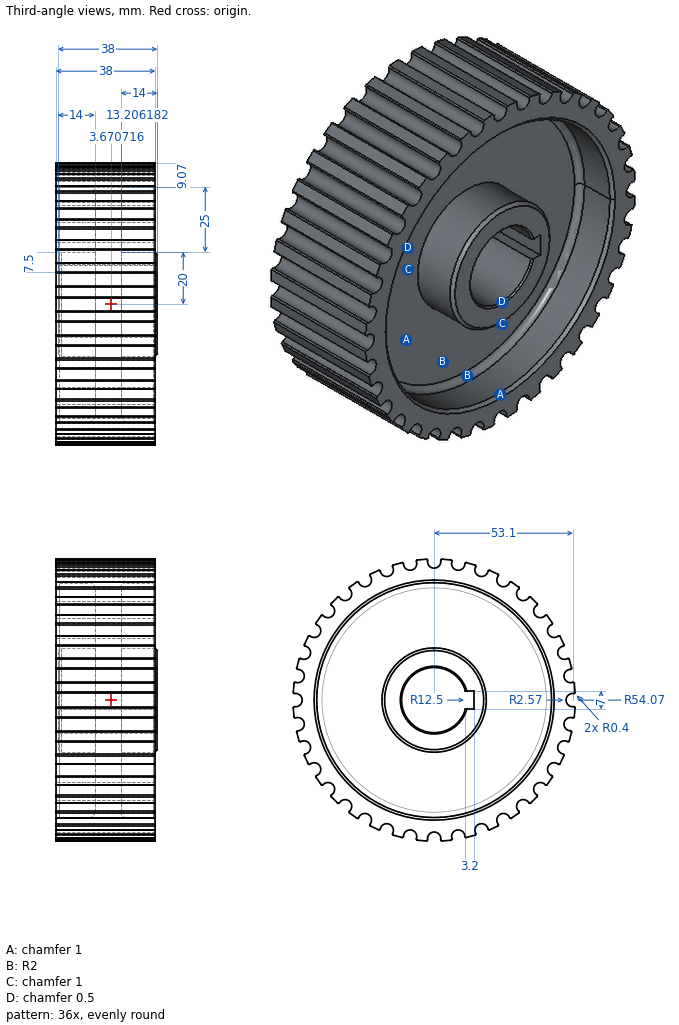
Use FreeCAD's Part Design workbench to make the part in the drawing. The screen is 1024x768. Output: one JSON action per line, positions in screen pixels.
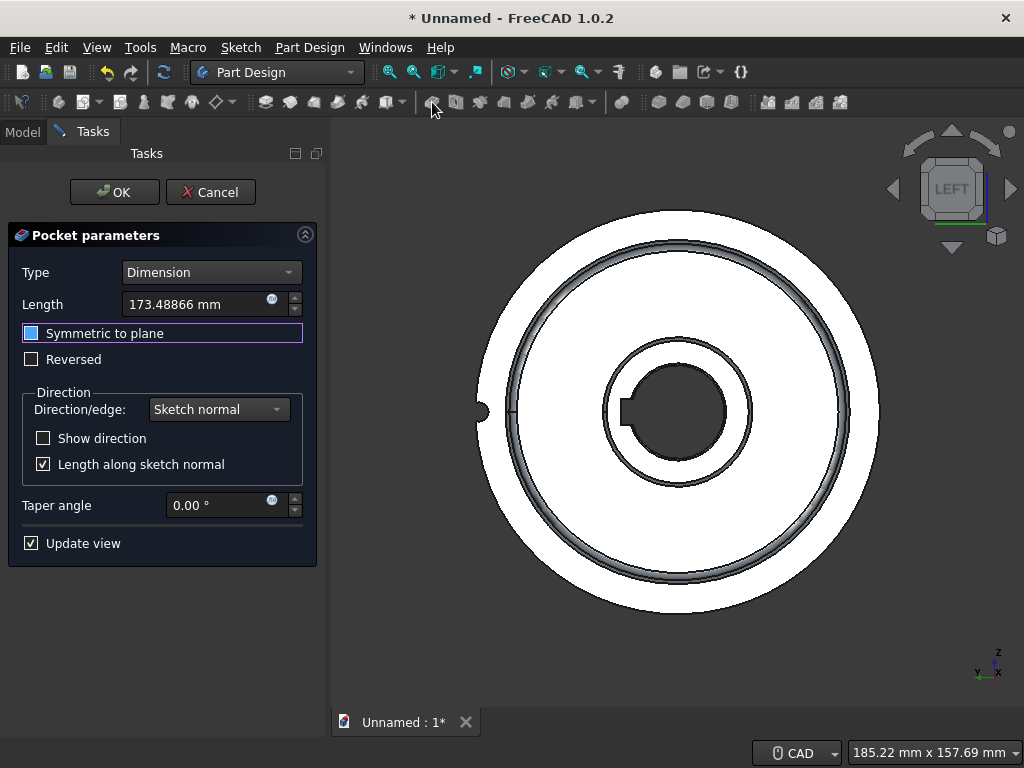
{"action": "left_click", "coordinate": [30, 333]}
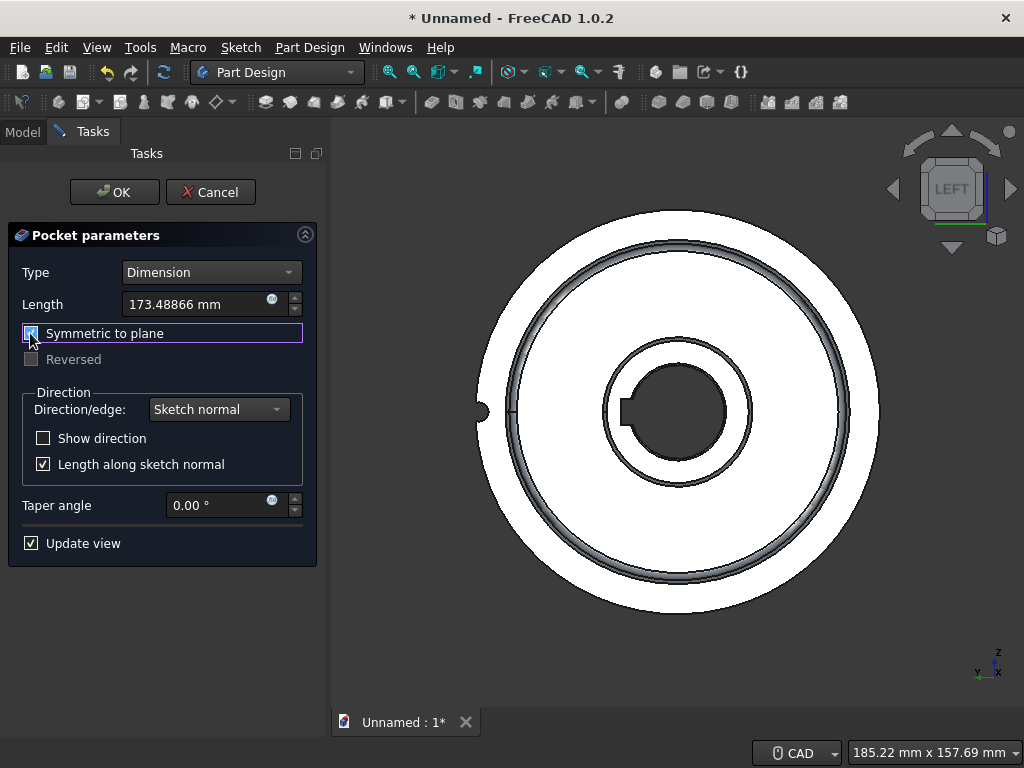
{"action": "left_click", "coordinate": [115, 192]}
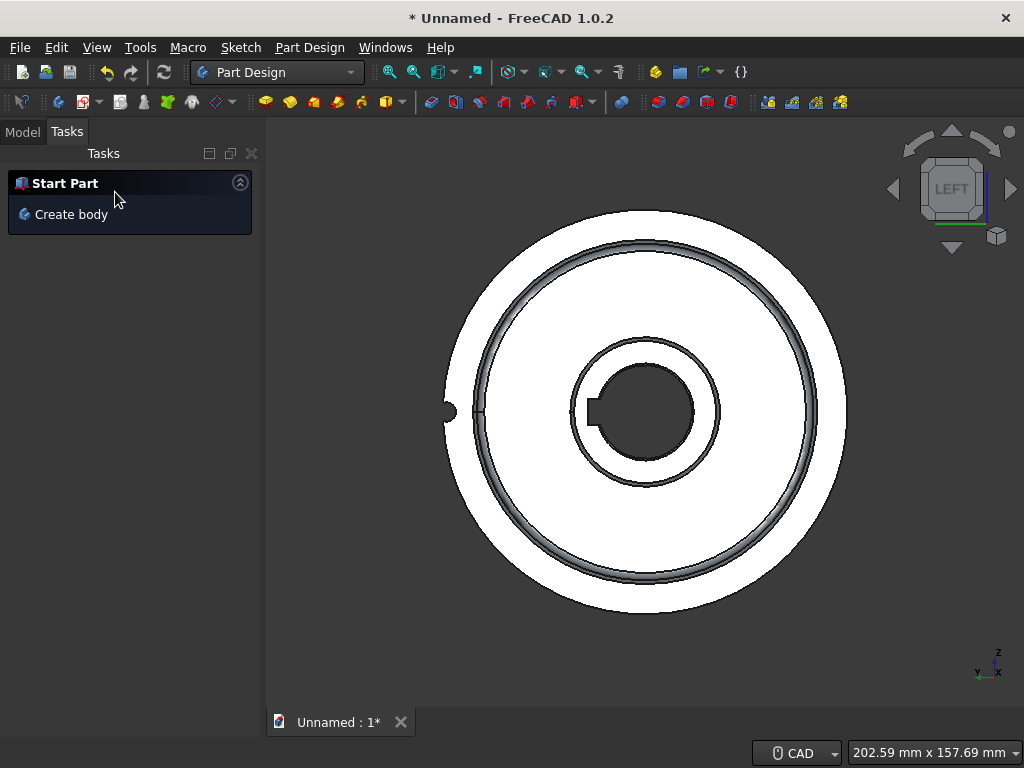
{"action": "left_click", "coordinate": [23, 131]}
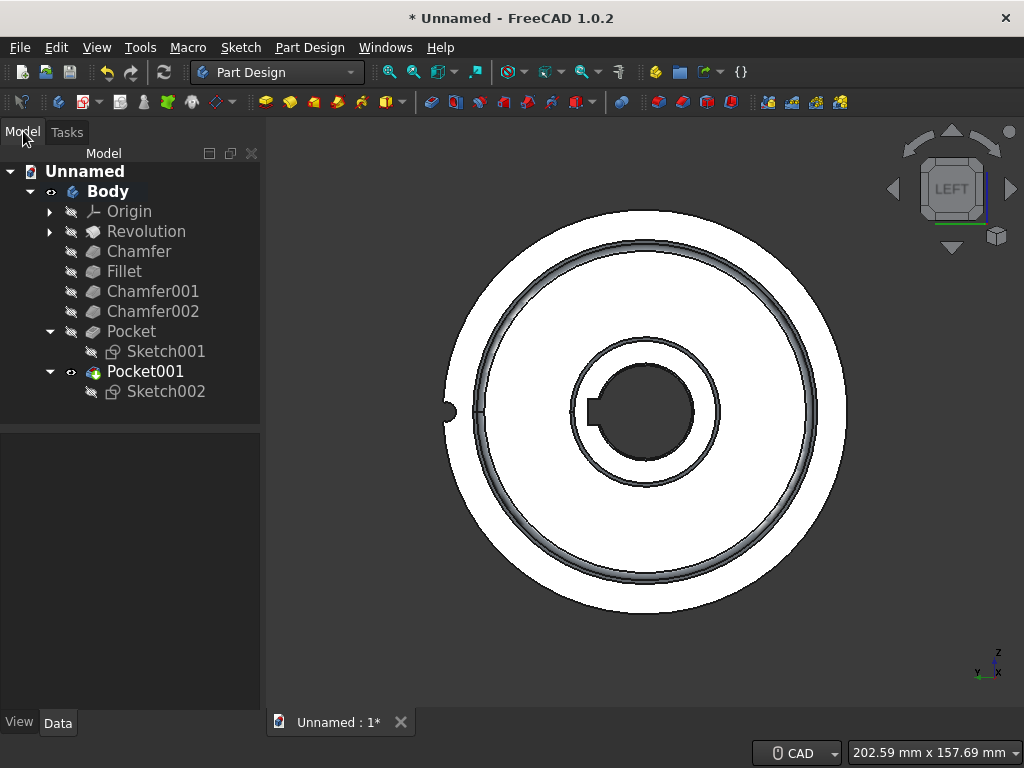
{"action": "left_click", "coordinate": [116, 372]}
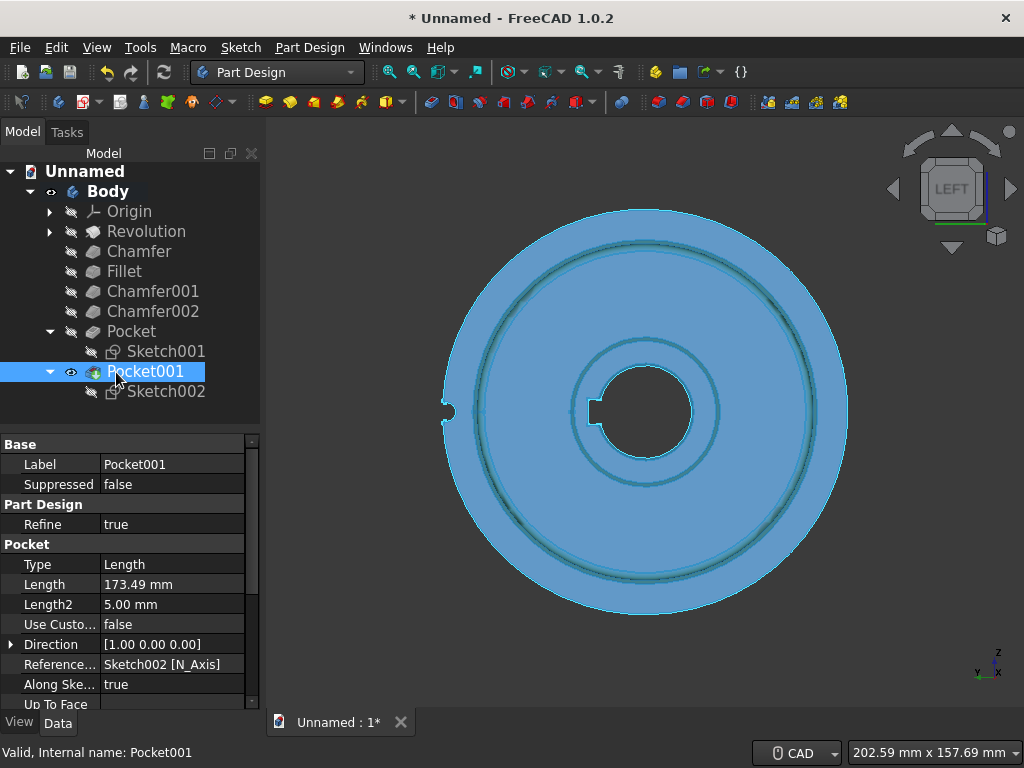
{"action": "left_click", "coordinate": [816, 102]}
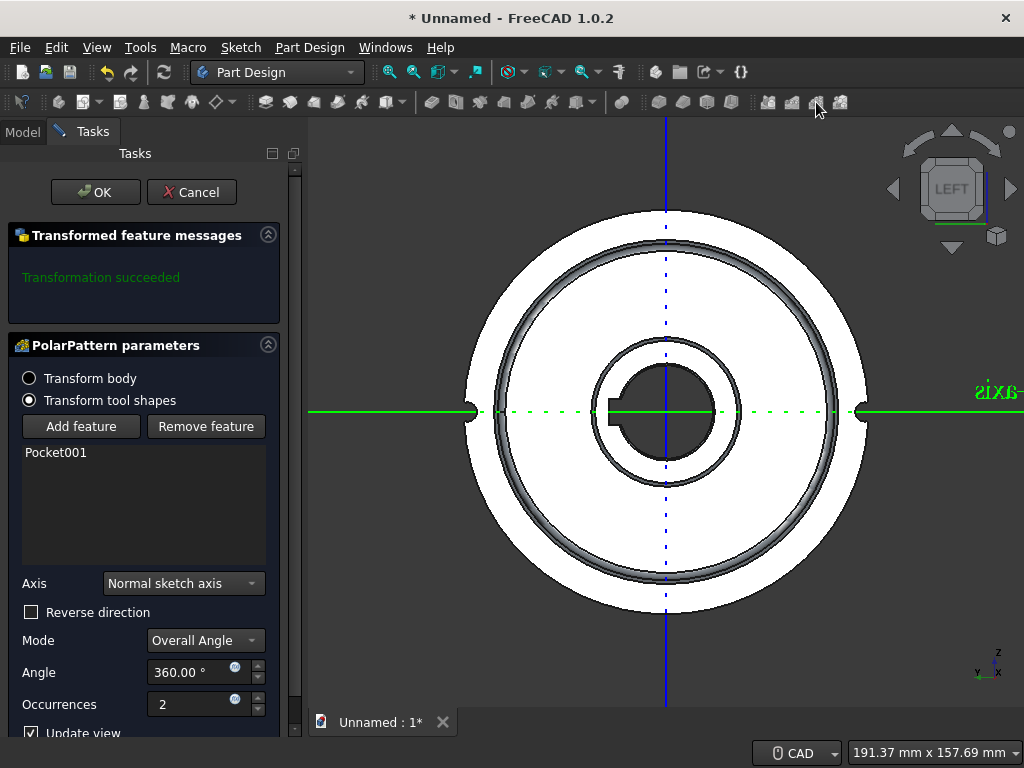
{"action": "left_click", "coordinate": [184, 584]}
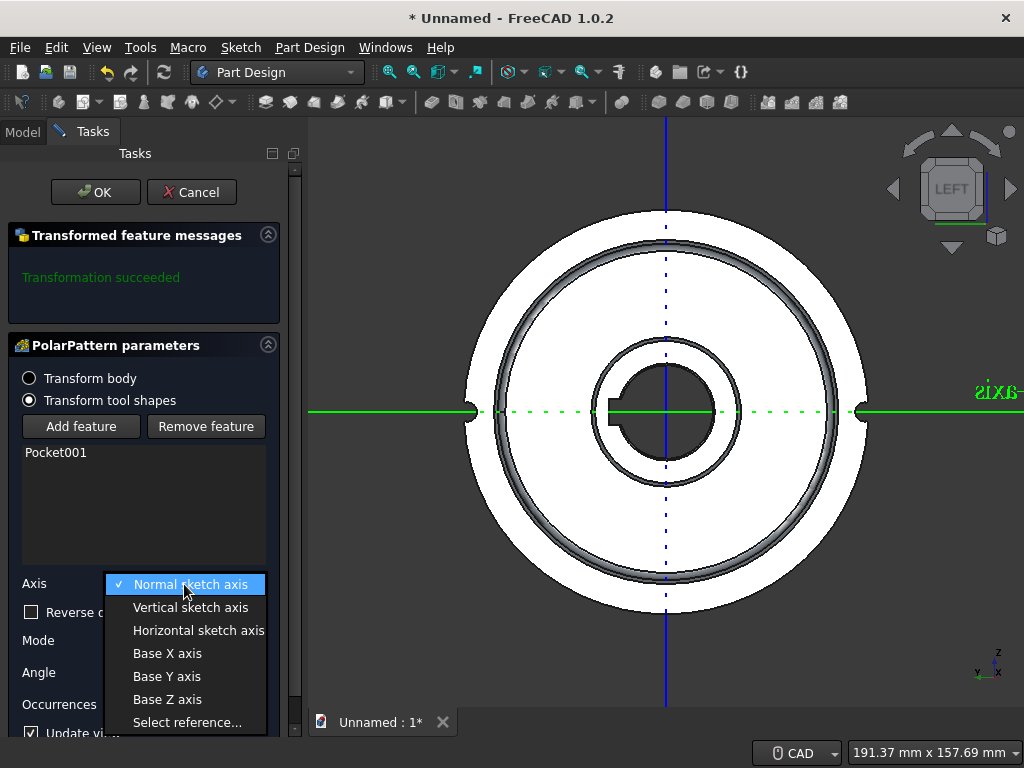
{"action": "left_click", "coordinate": [184, 654]}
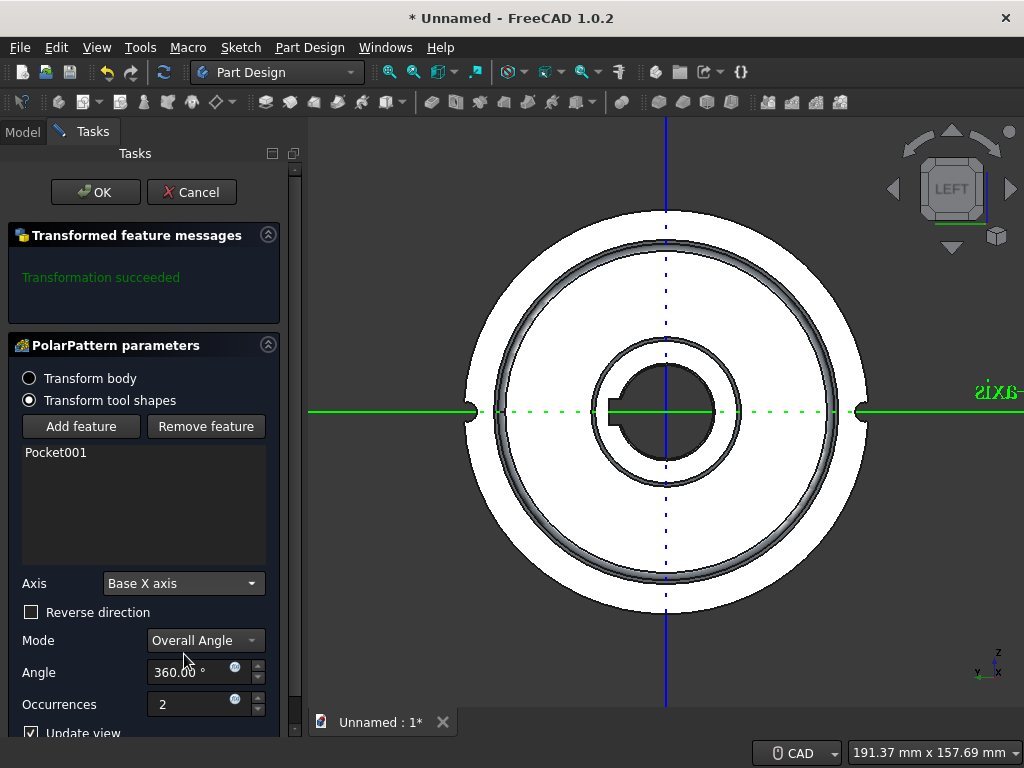
{"action": "triple_click", "coordinate": [198, 704]}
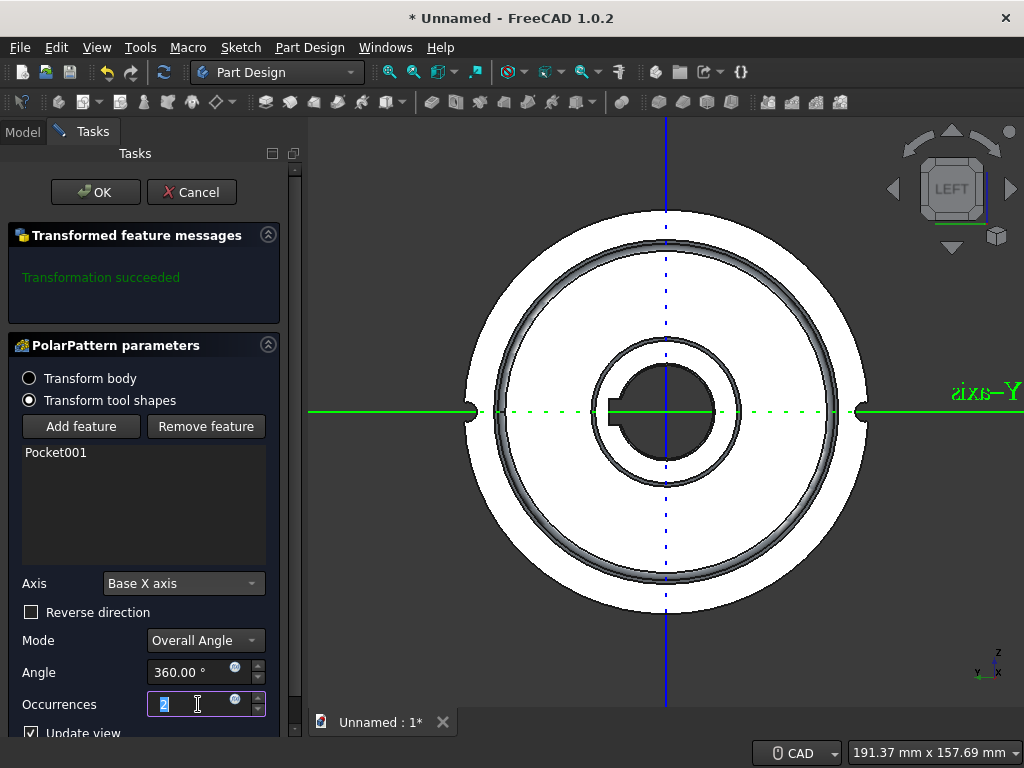
{"action": "type", "text": "36"}
{"action": "key", "text": "Tab"}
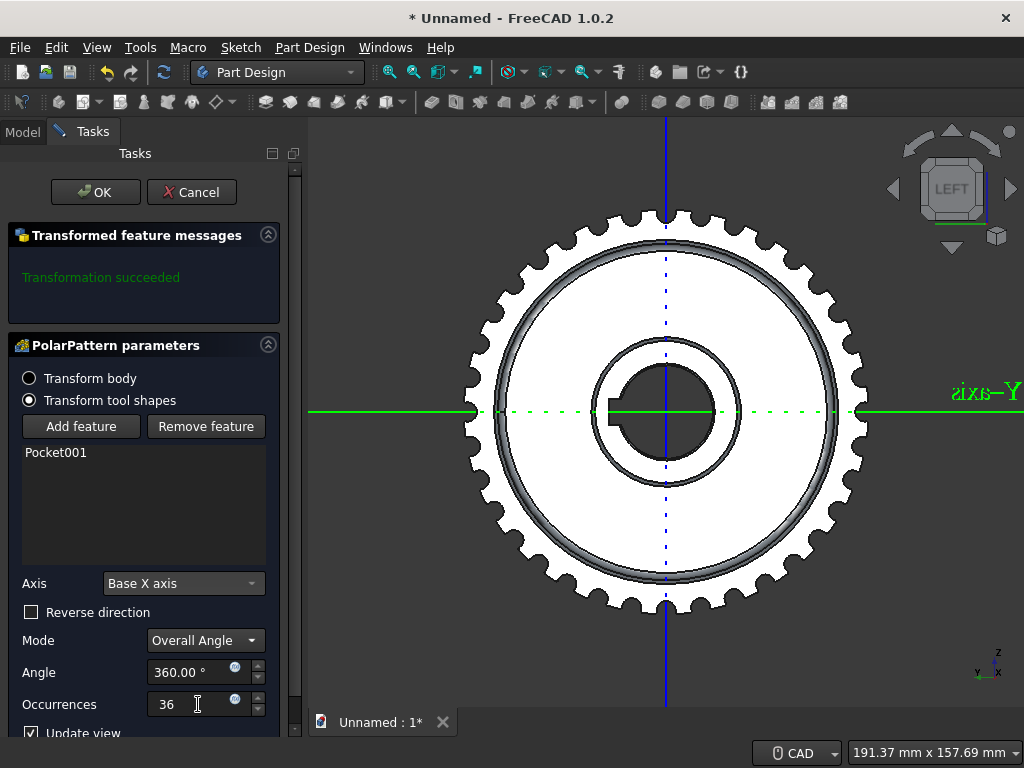
{"action": "left_click", "coordinate": [96, 192]}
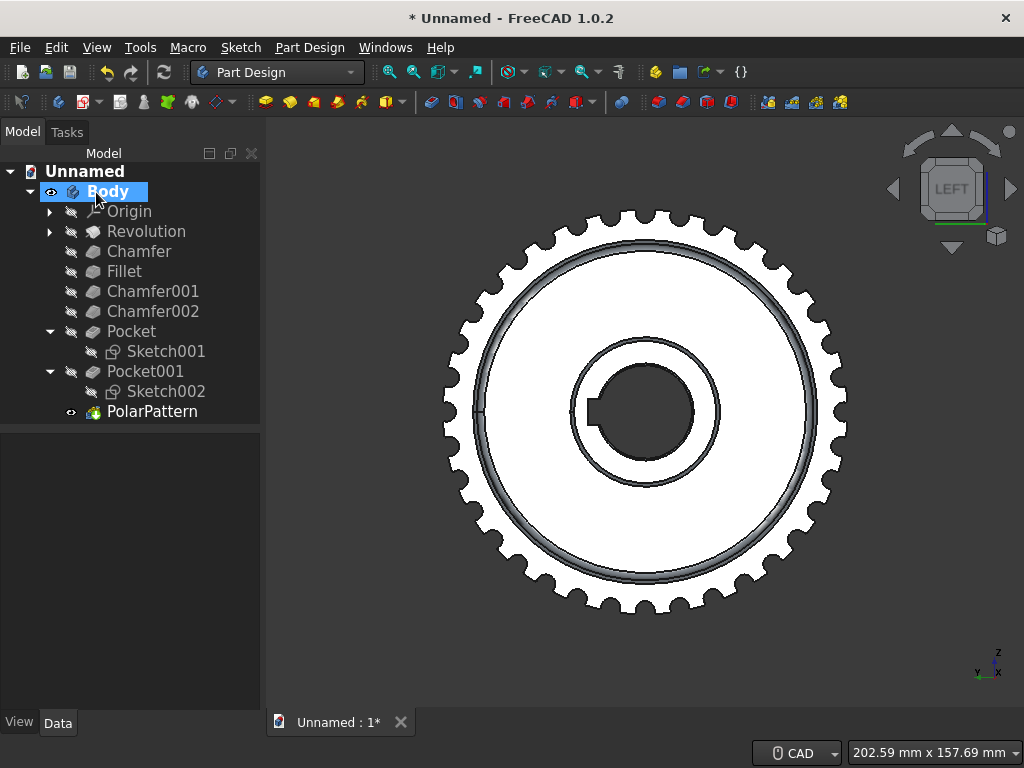
{"action": "key", "text": "0"}